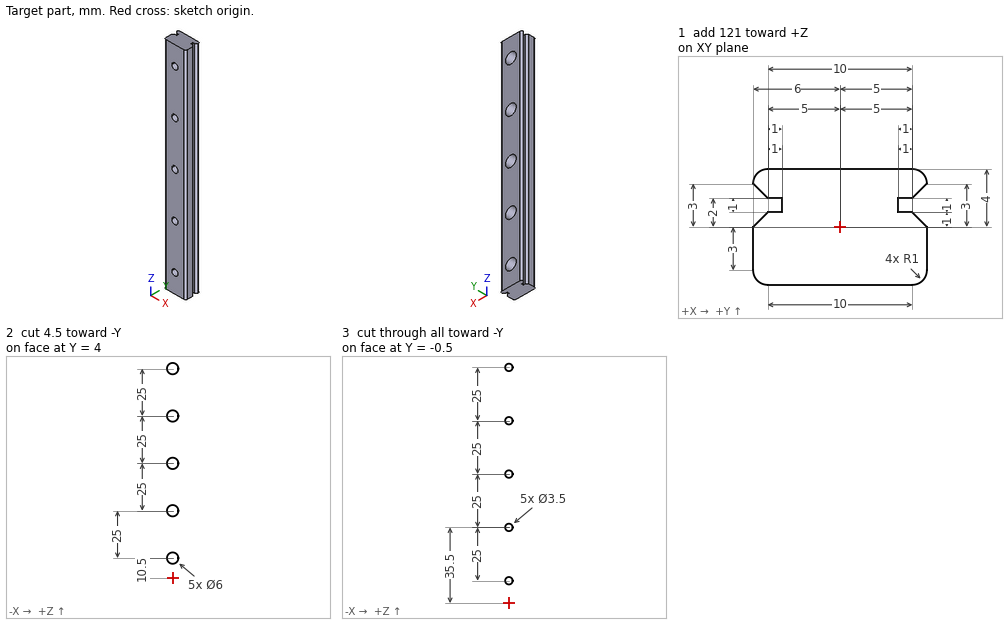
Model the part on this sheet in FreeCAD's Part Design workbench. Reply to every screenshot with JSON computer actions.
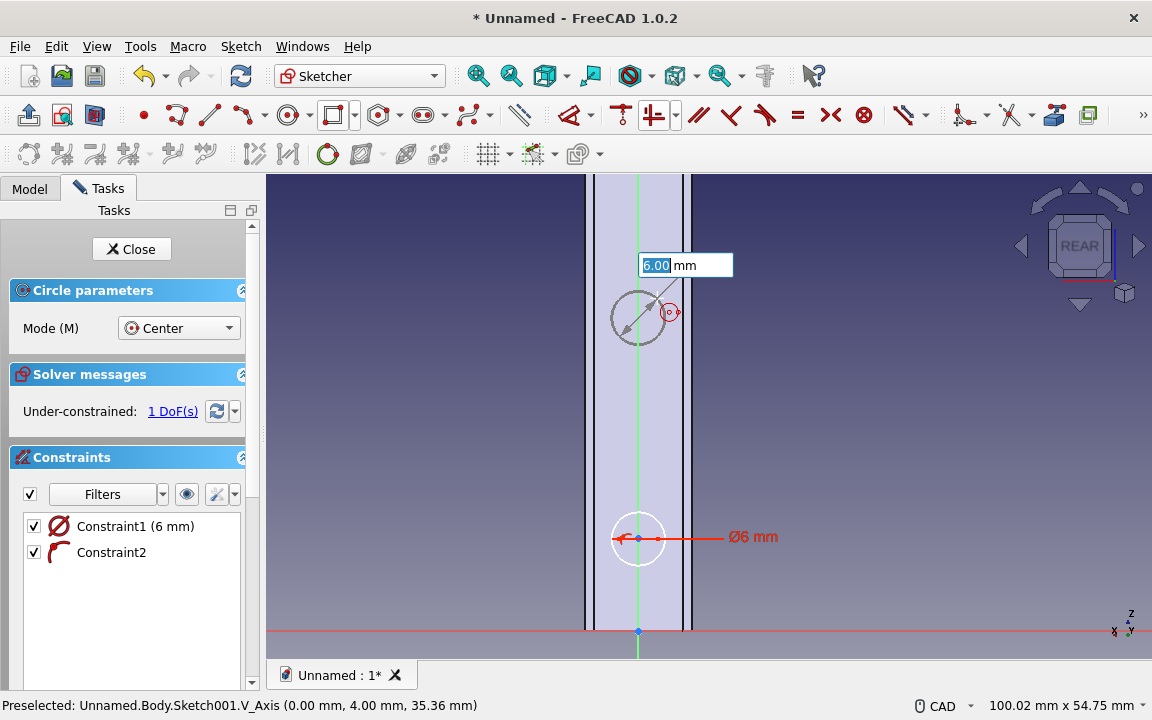
{"action": "type", "text": "6"}
{"action": "key", "text": "Return"}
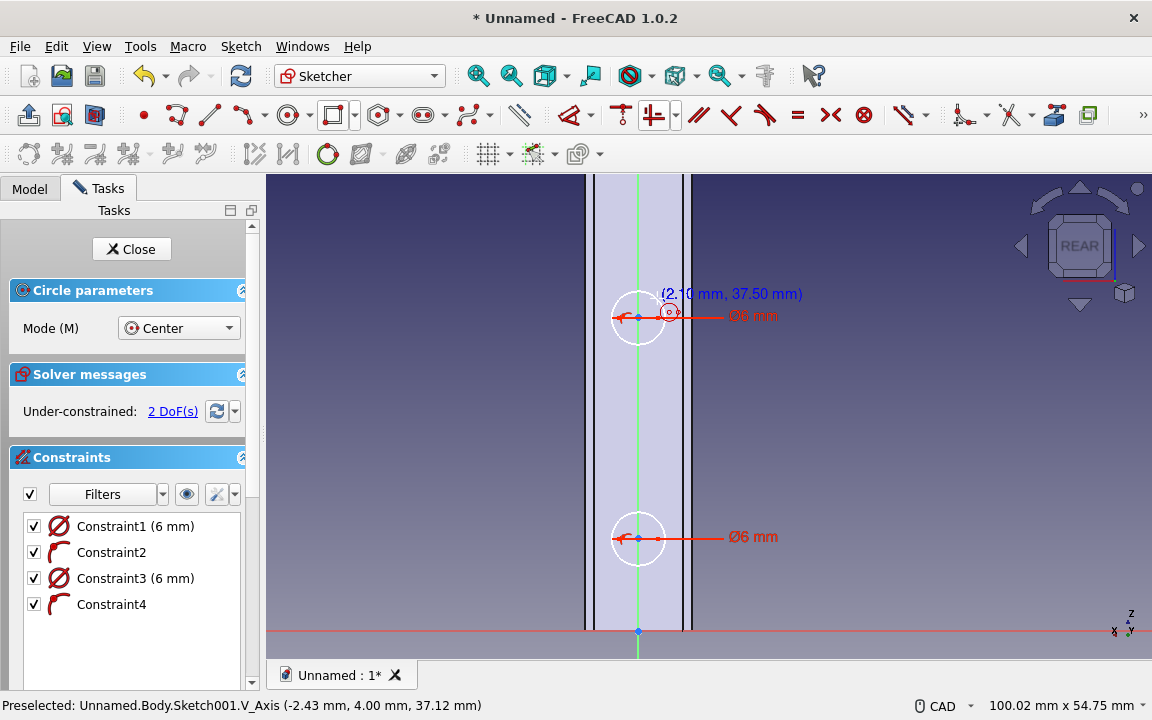
{"action": "scroll", "coordinate": [641, 541], "scroll_direction": "down", "scroll_amount": 6}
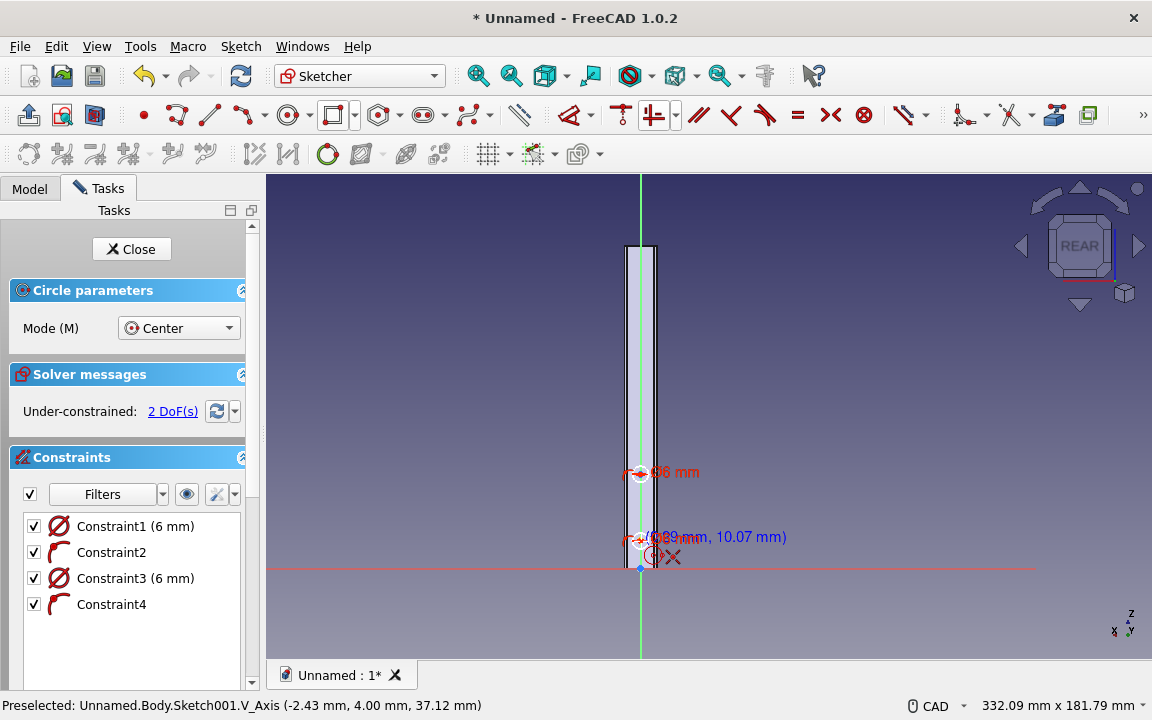
{"action": "scroll", "coordinate": [641, 407], "scroll_direction": "up", "scroll_amount": 6}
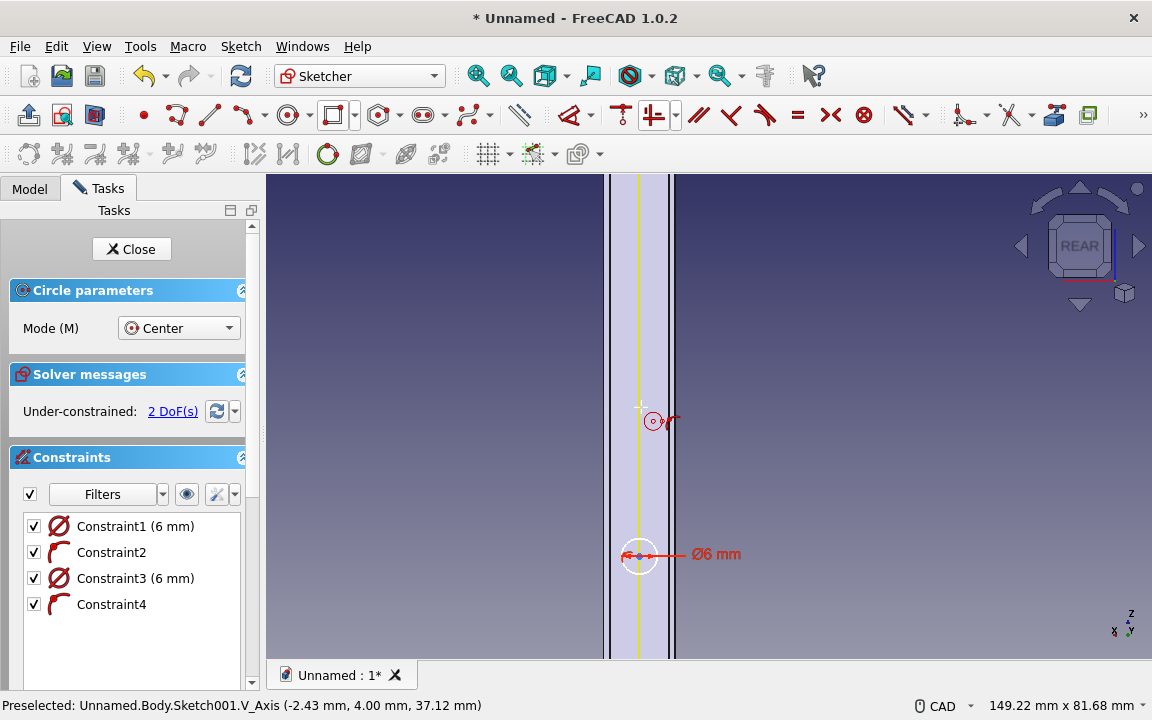
{"action": "left_click", "coordinate": [638, 407]}
{"action": "mouse_move", "coordinate": [657, 388]}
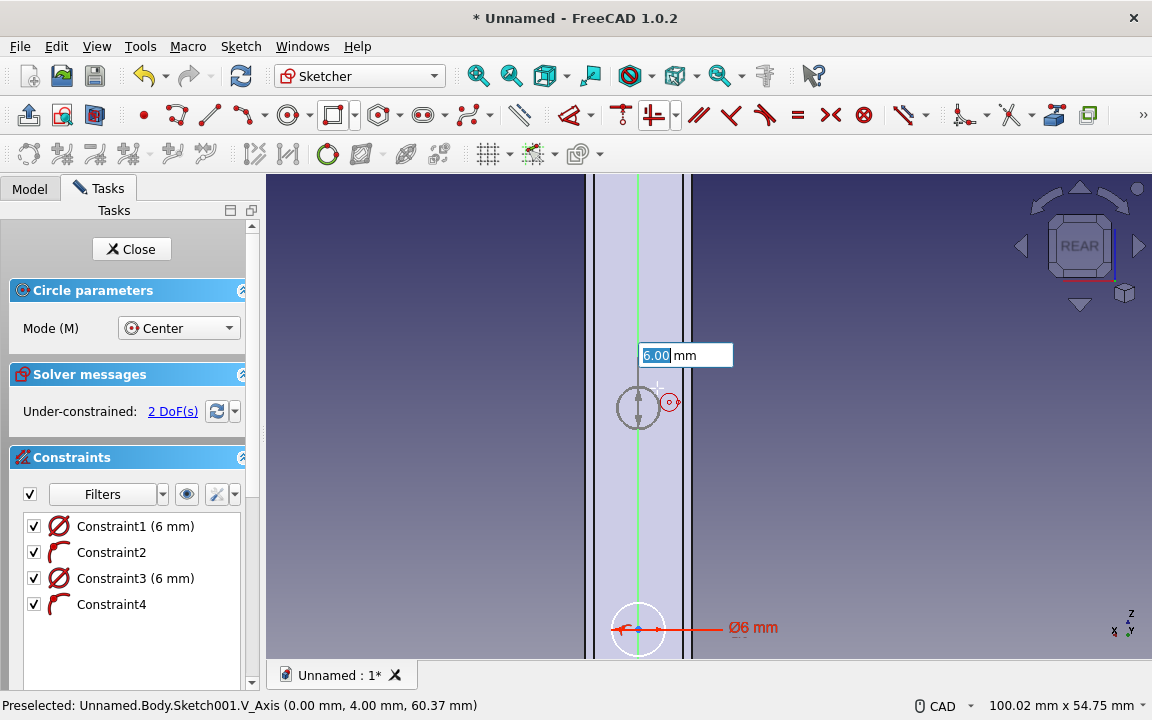
{"action": "type", "text": "6"}
{"action": "key", "text": "Return"}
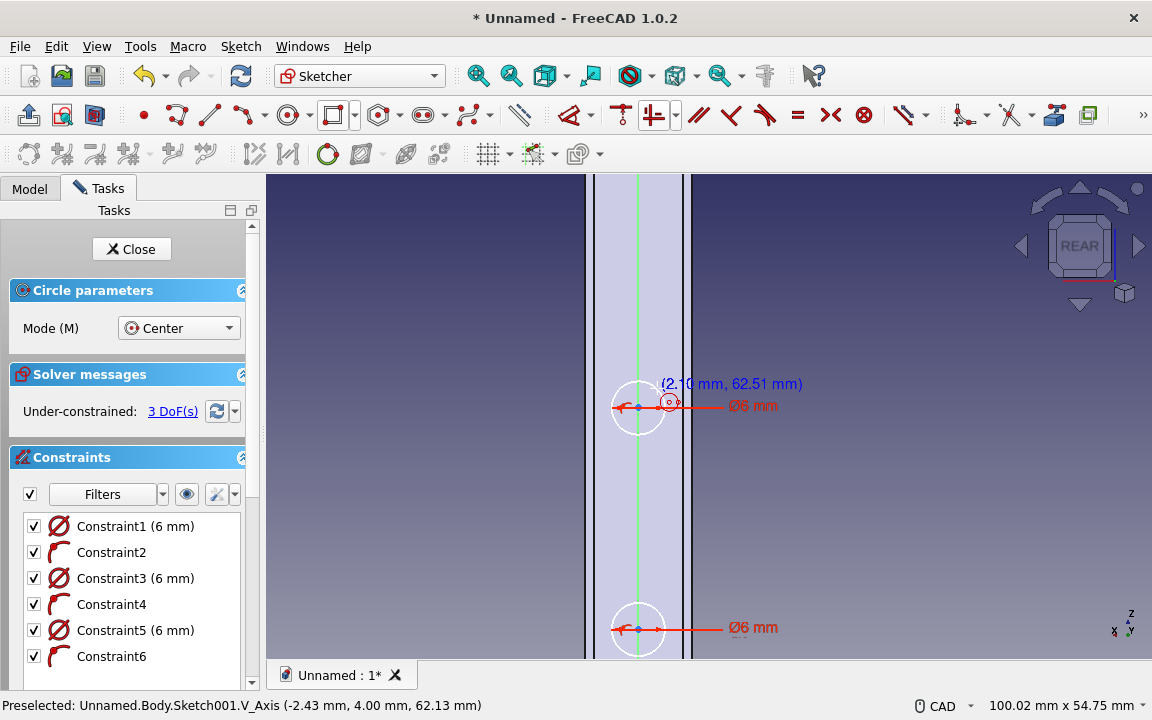
{"action": "scroll", "coordinate": [641, 406], "scroll_direction": "down", "scroll_amount": 6}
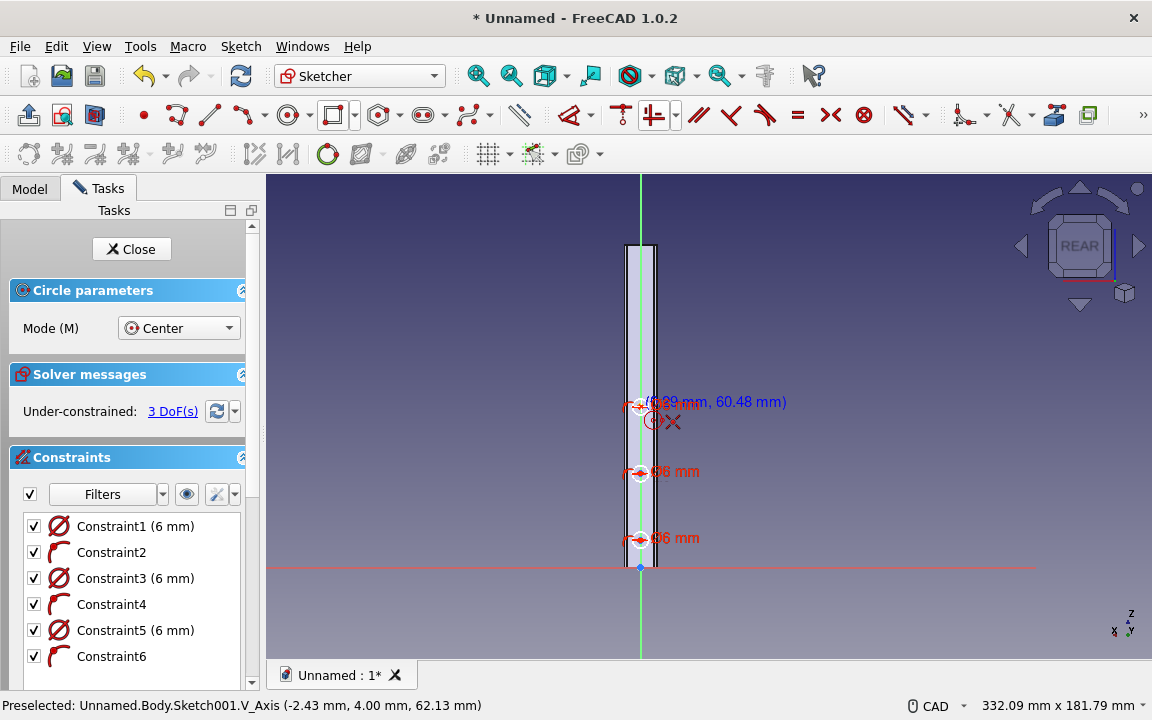
{"action": "scroll", "coordinate": [641, 340], "scroll_direction": "up", "scroll_amount": 6}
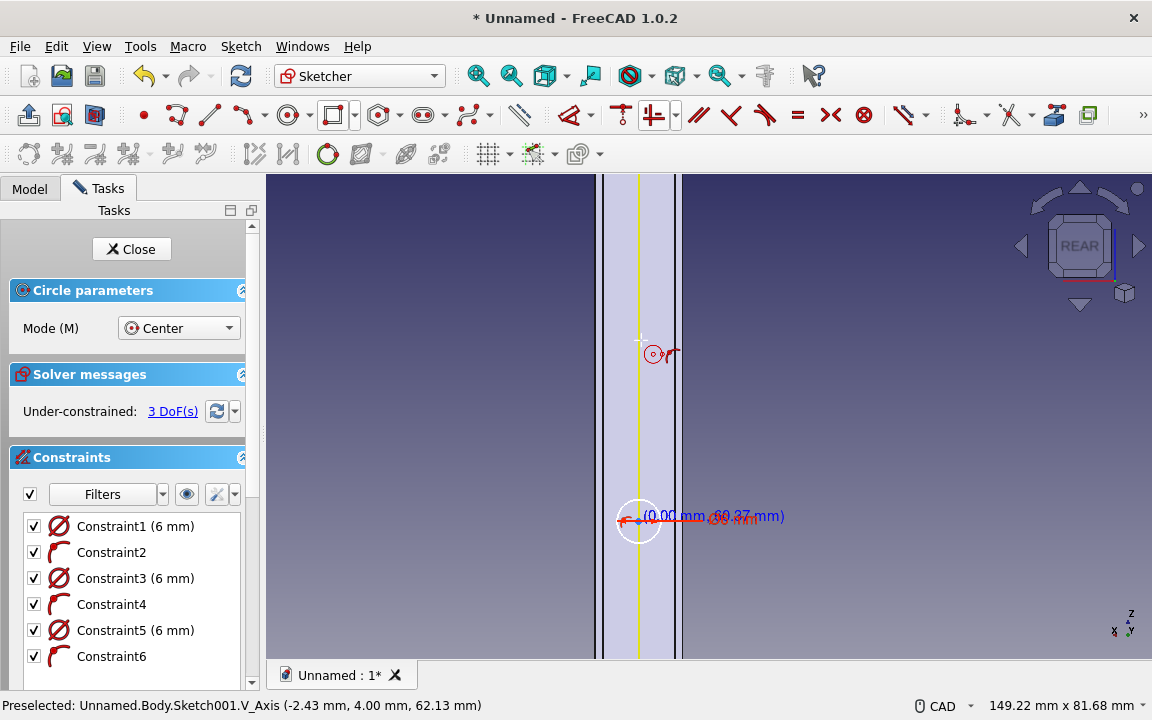
{"action": "left_click", "coordinate": [638, 339]}
{"action": "mouse_move", "coordinate": [657, 320]}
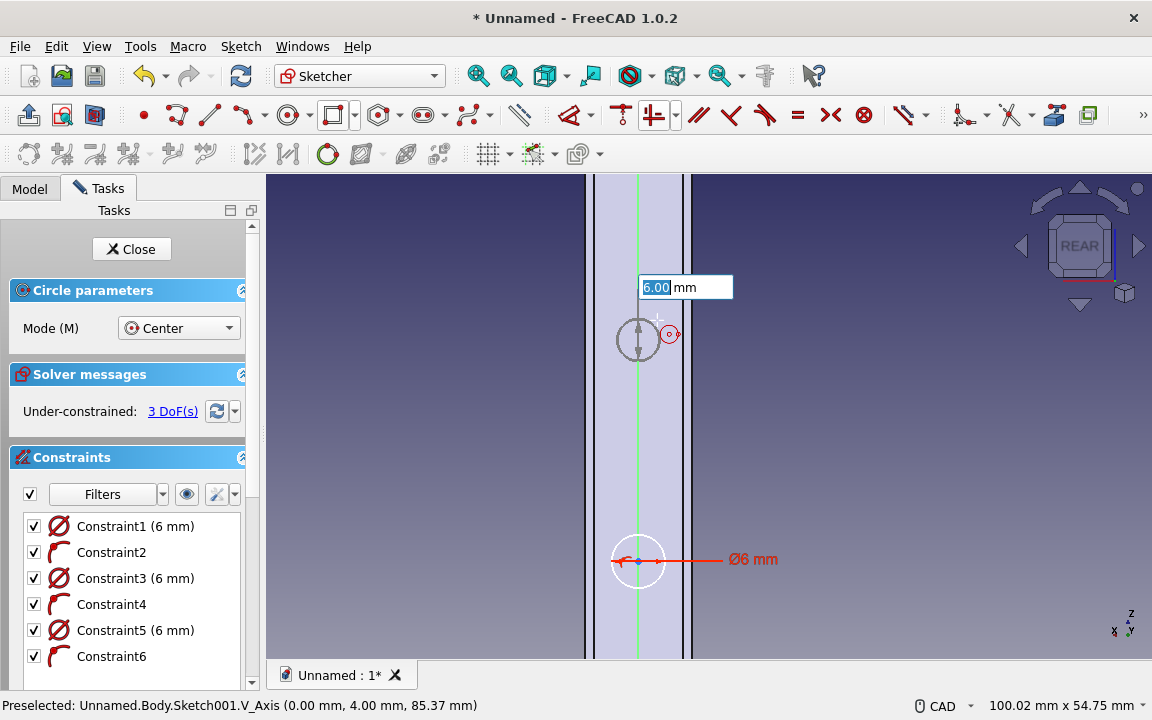
{"action": "type", "text": "6"}
{"action": "key", "text": "Return"}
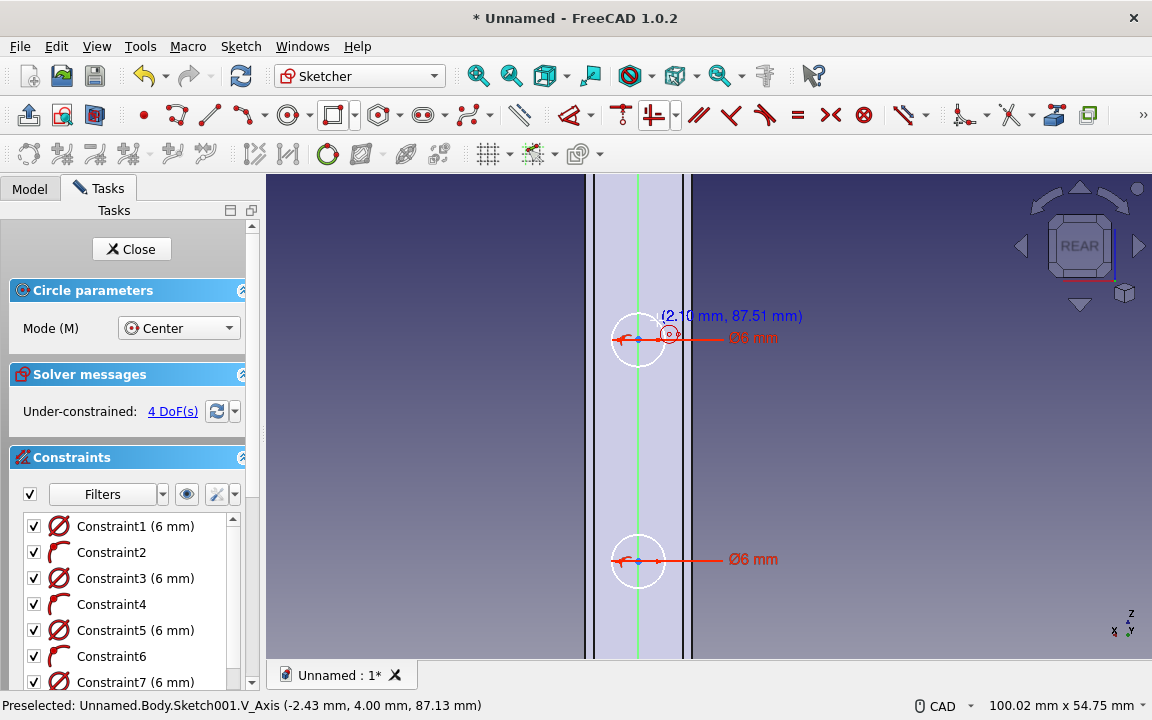
{"action": "scroll", "coordinate": [641, 340], "scroll_direction": "down", "scroll_amount": 6}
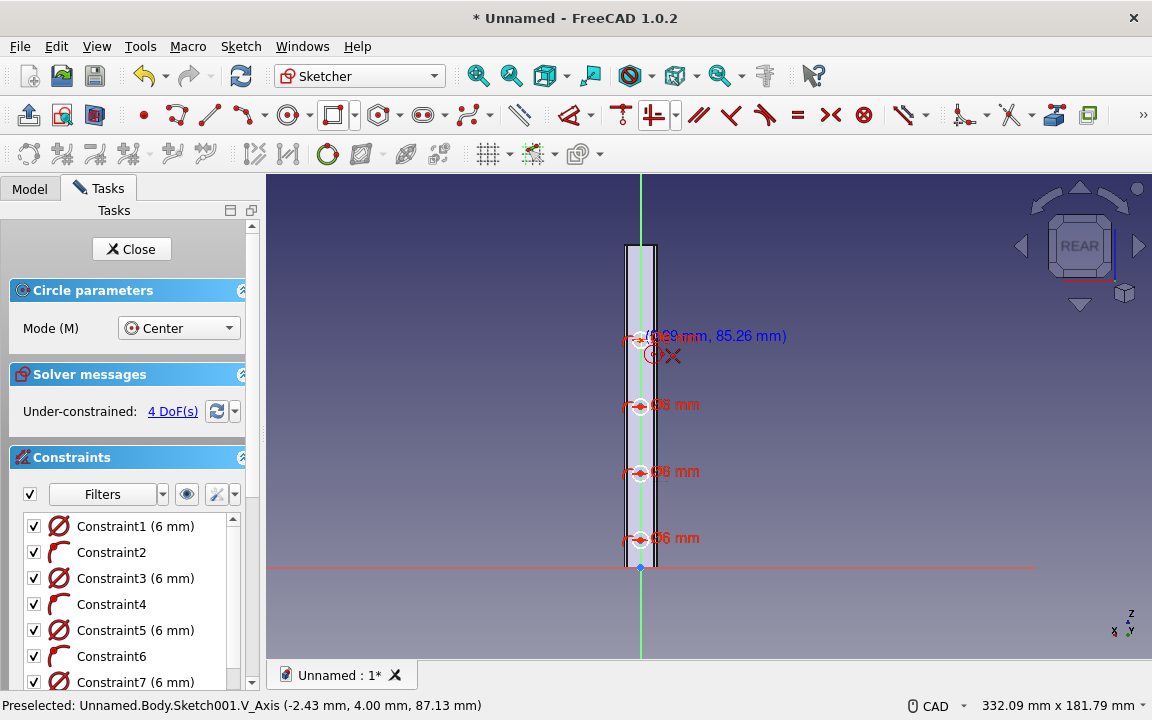
{"action": "scroll", "coordinate": [641, 273], "scroll_direction": "up", "scroll_amount": 6}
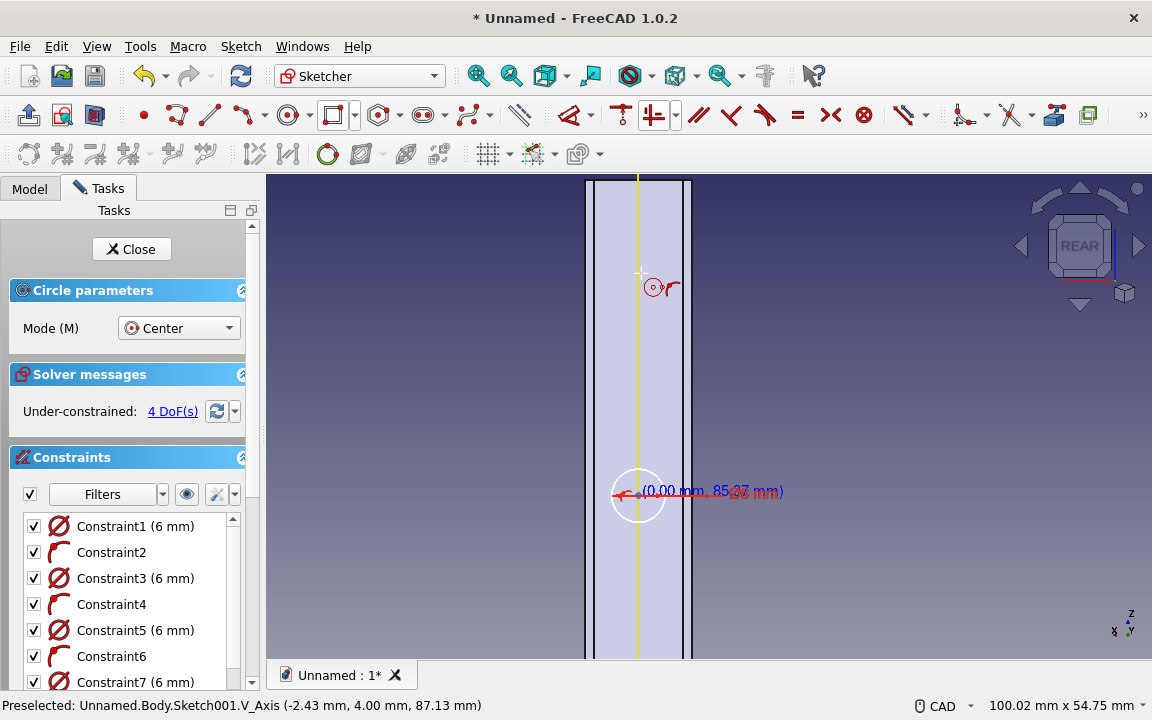
{"action": "left_click", "coordinate": [638, 273]}
{"action": "mouse_move", "coordinate": [657, 254]}